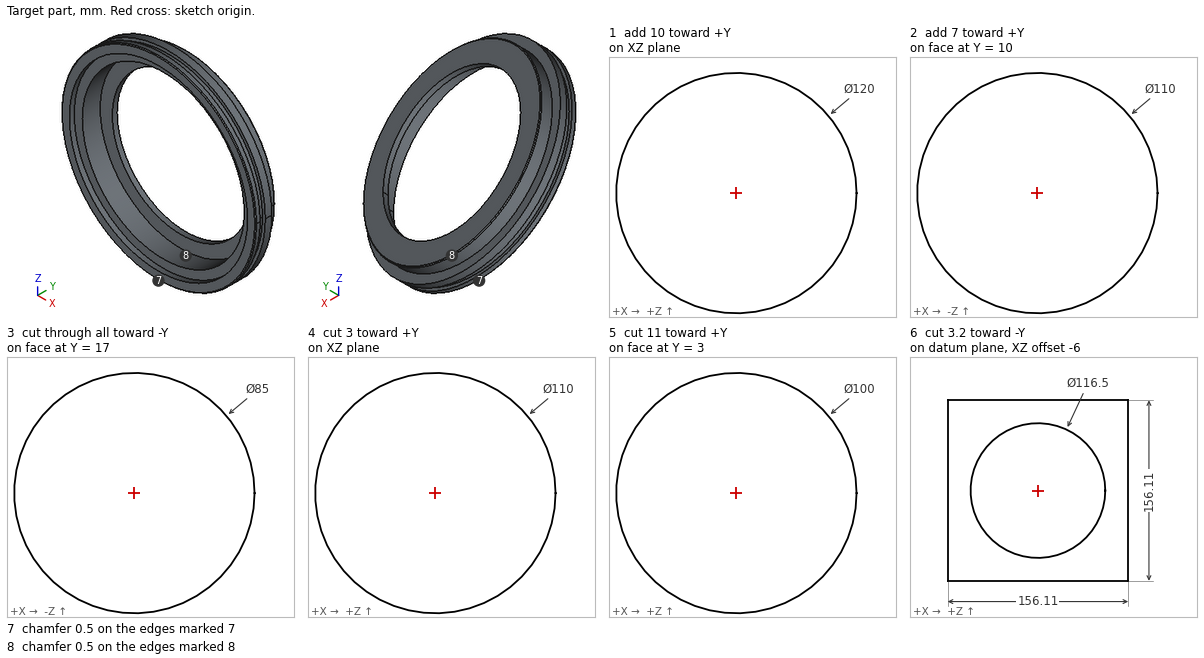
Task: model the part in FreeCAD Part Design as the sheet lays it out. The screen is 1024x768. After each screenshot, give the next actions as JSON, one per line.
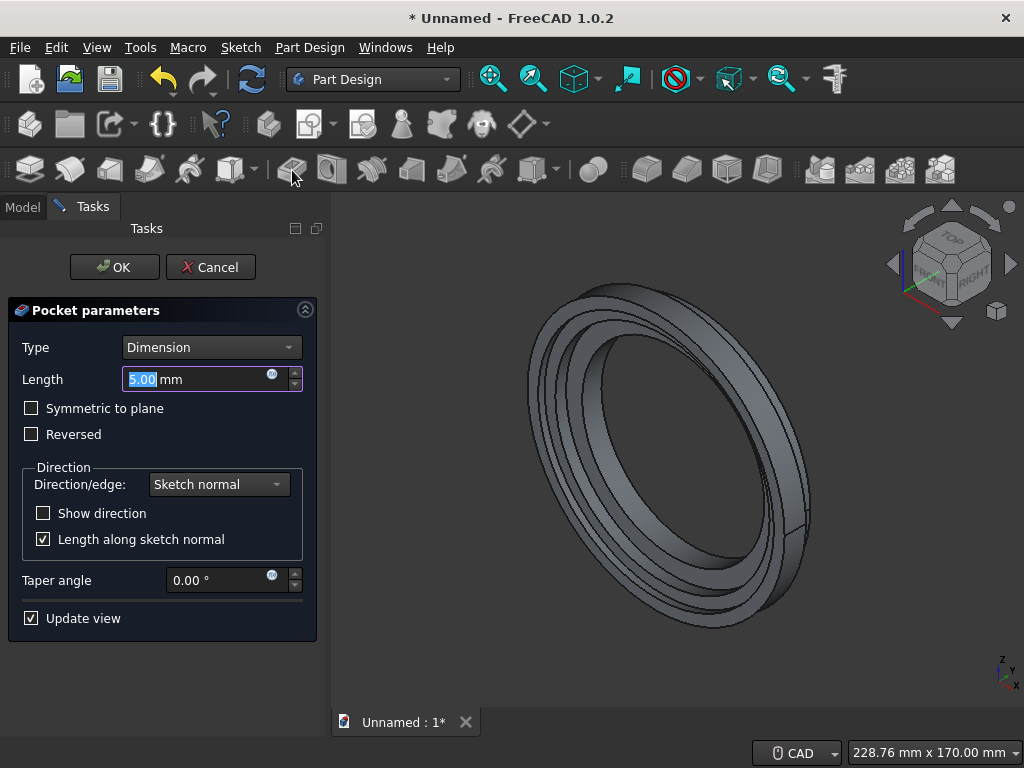
{"action": "type", "text": "11"}
{"action": "key", "text": "Tab"}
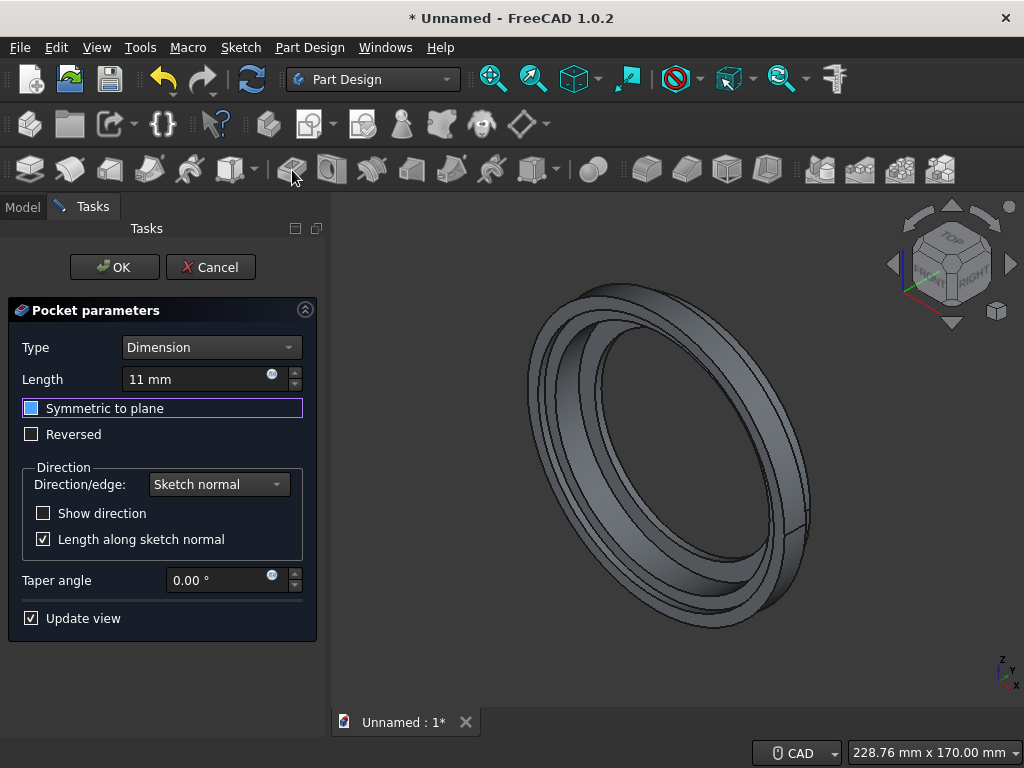
{"action": "left_click", "coordinate": [115, 267]}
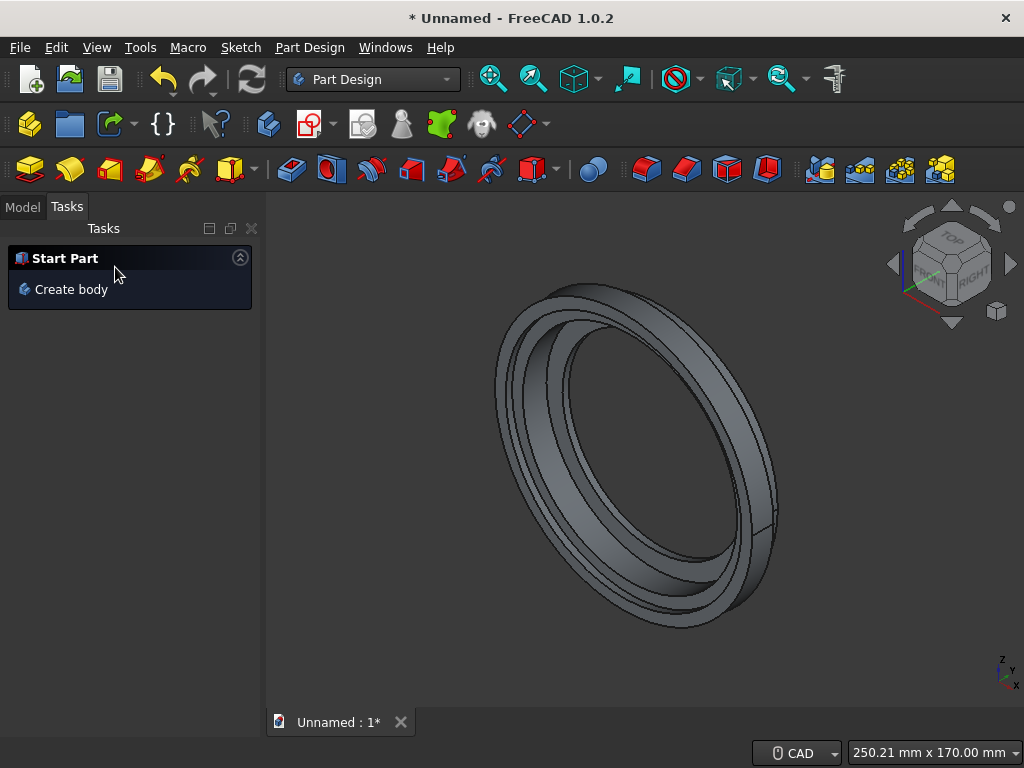
{"action": "left_click", "coordinate": [23, 206]}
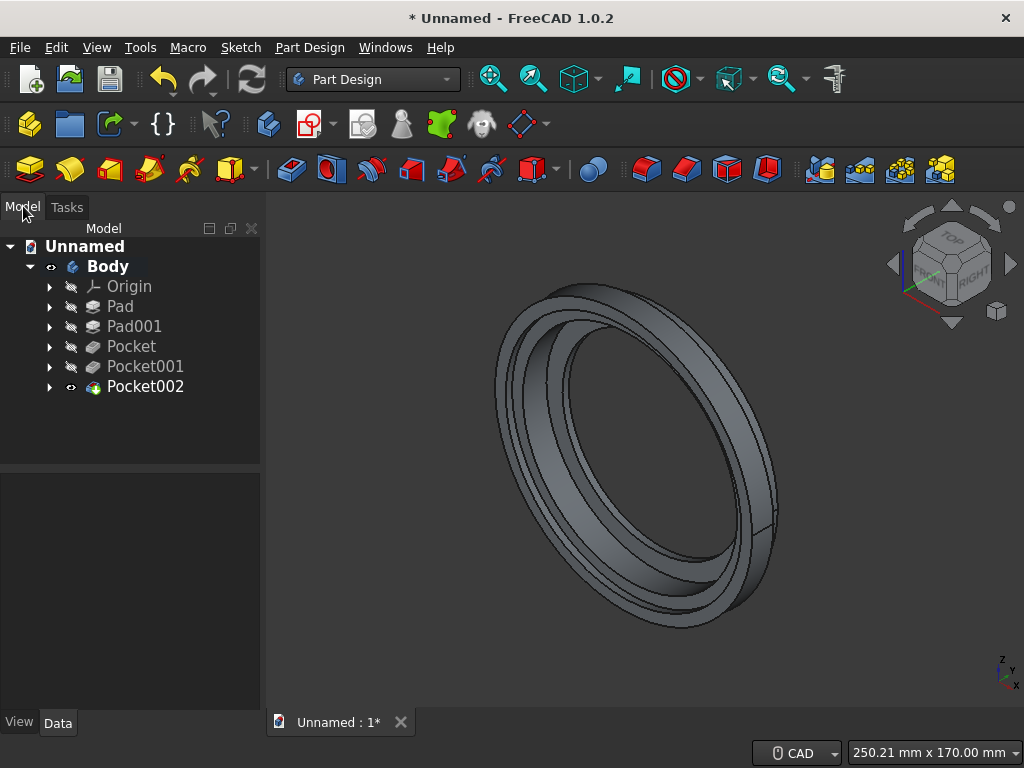
{"action": "left_click", "coordinate": [50, 287]}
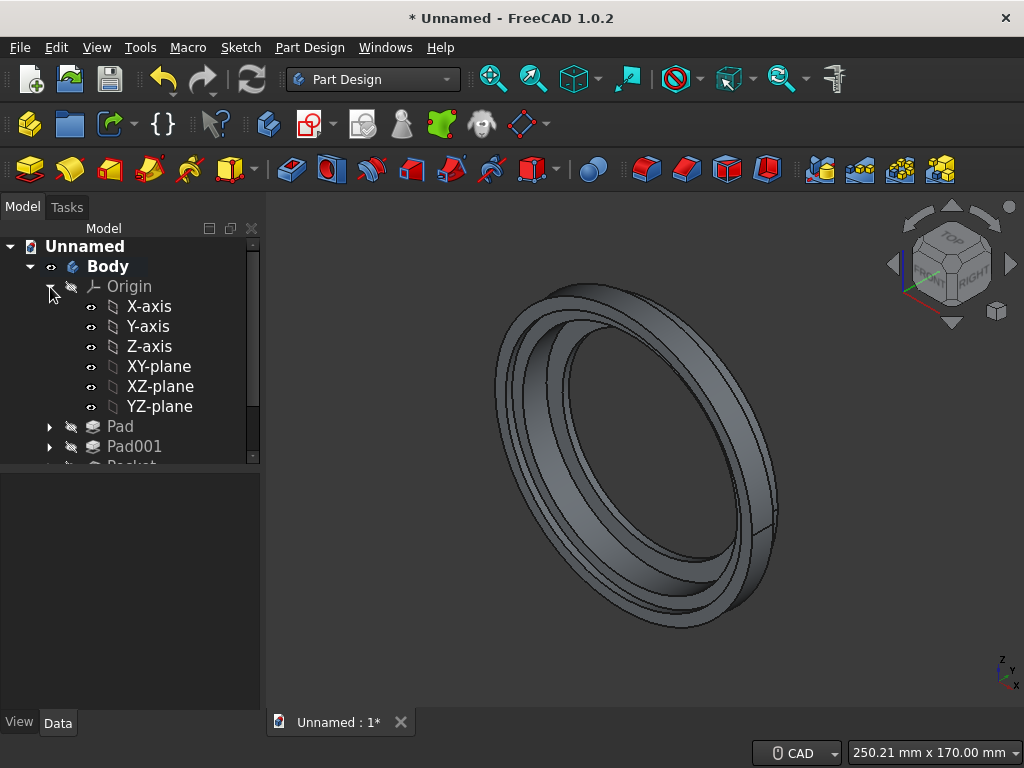
{"action": "left_click", "coordinate": [136, 387]}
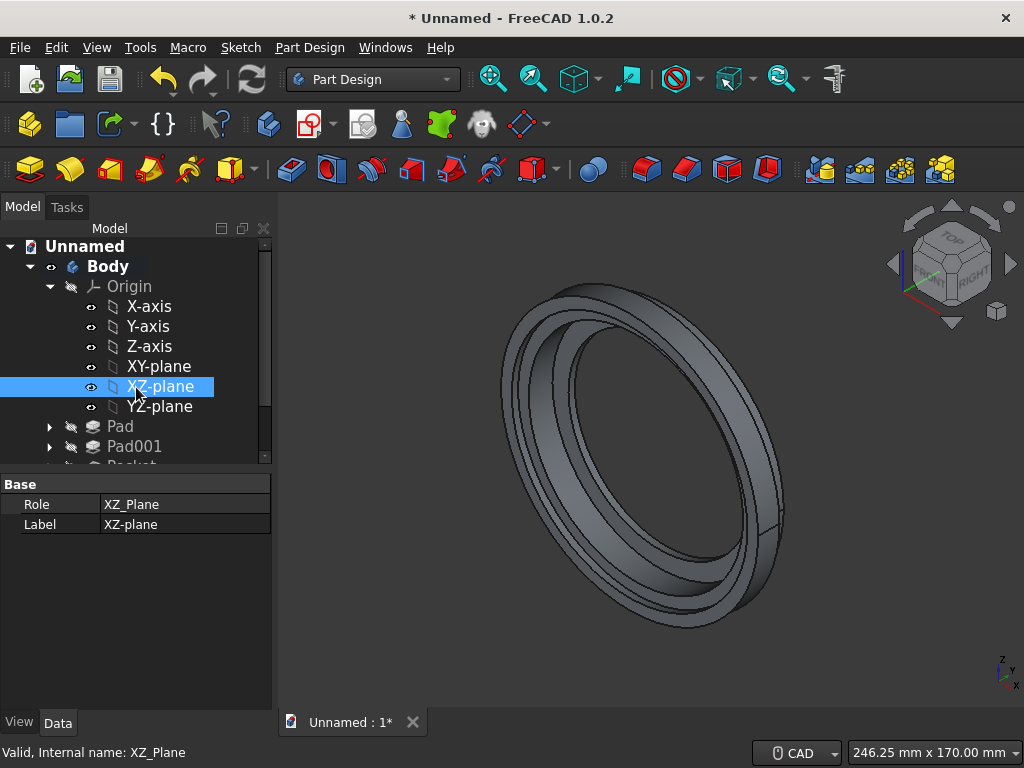
{"action": "left_click", "coordinate": [522, 124]}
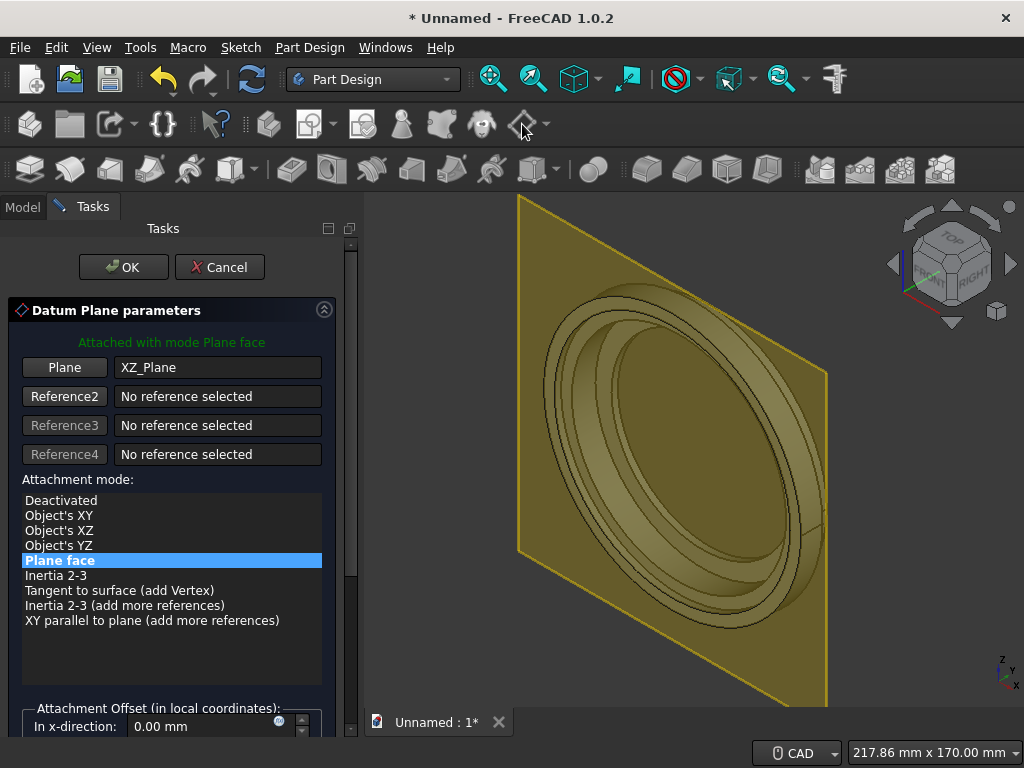
{"action": "scroll", "coordinate": [351, 487], "scroll_direction": "down", "scroll_amount": 3}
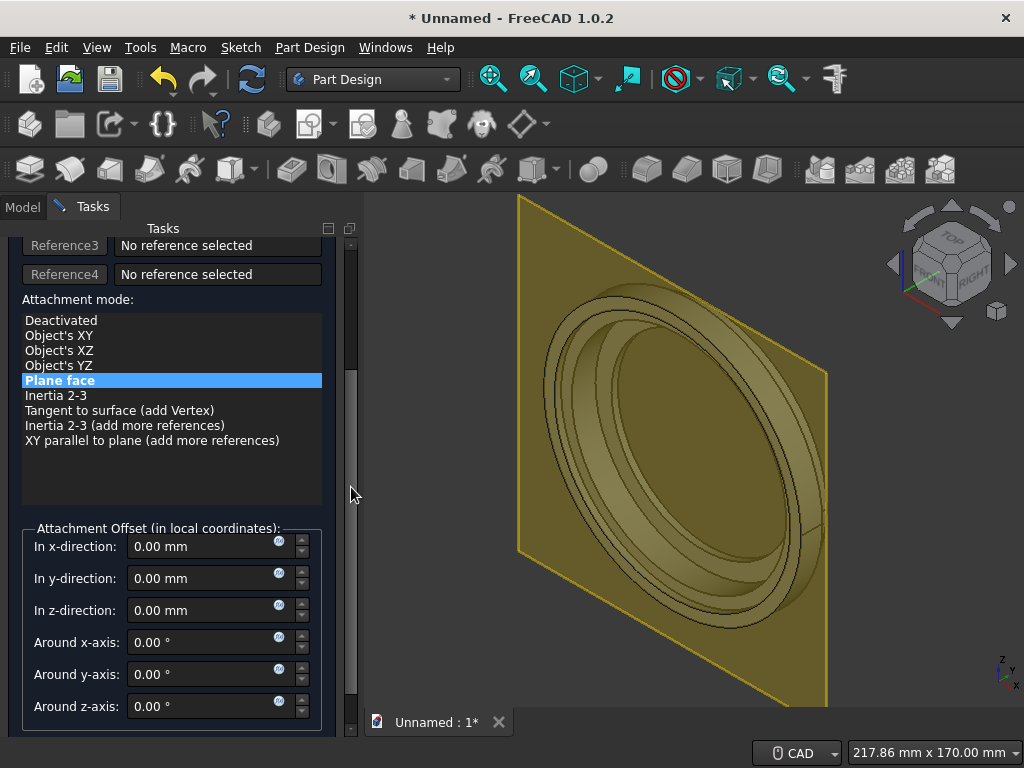
{"action": "triple_click", "coordinate": [210, 610]}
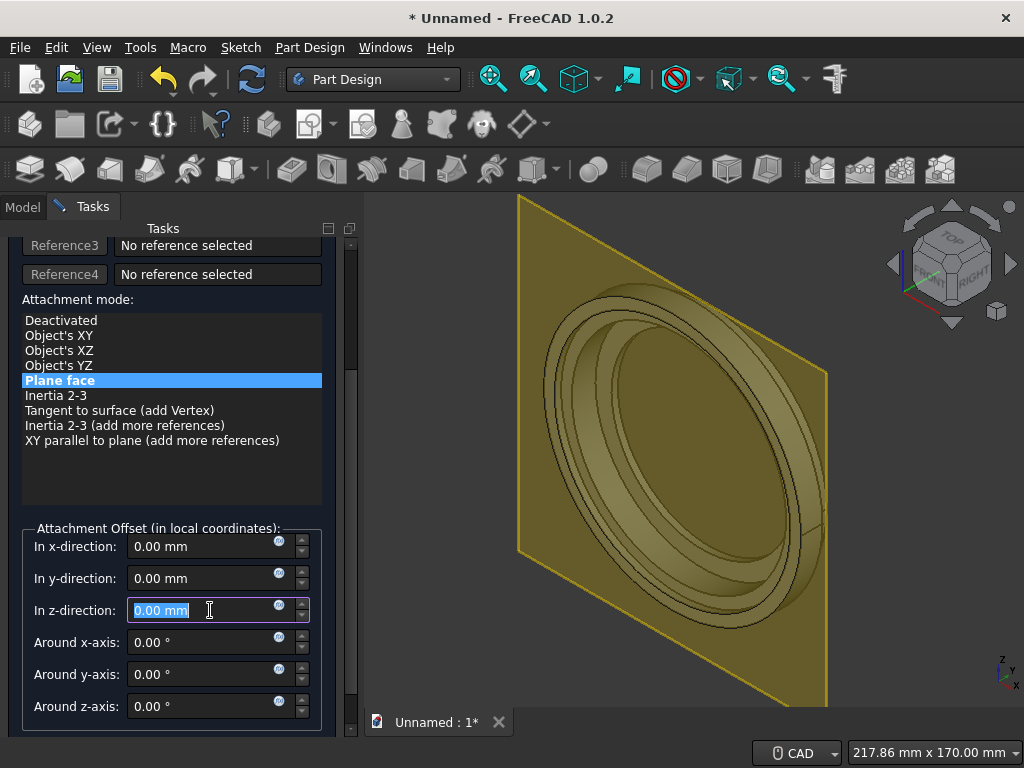
{"action": "type", "text": "-6"}
{"action": "key", "text": "Tab"}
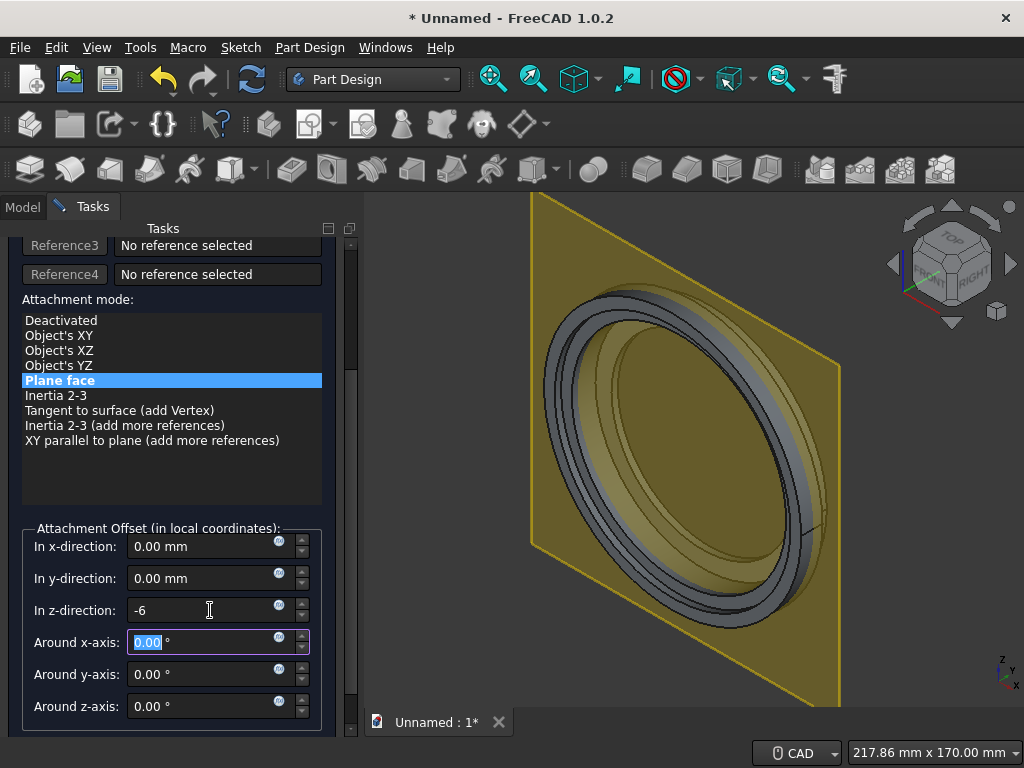
{"action": "scroll", "coordinate": [351, 487], "scroll_direction": "up", "scroll_amount": 4}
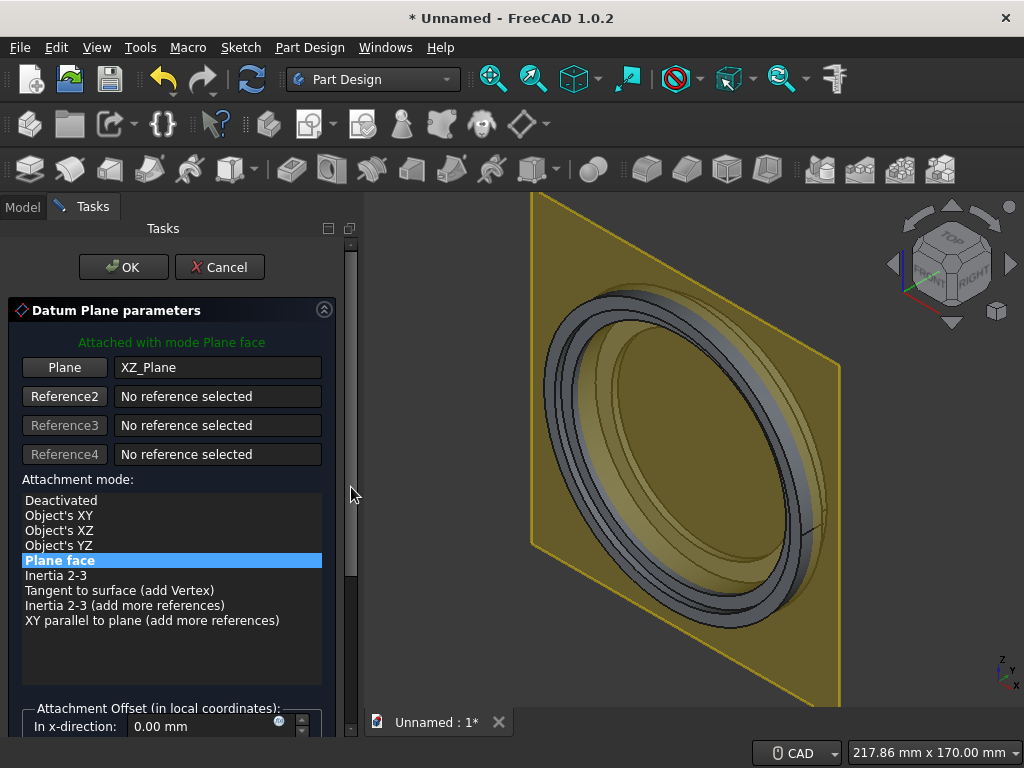
{"action": "left_click", "coordinate": [124, 267]}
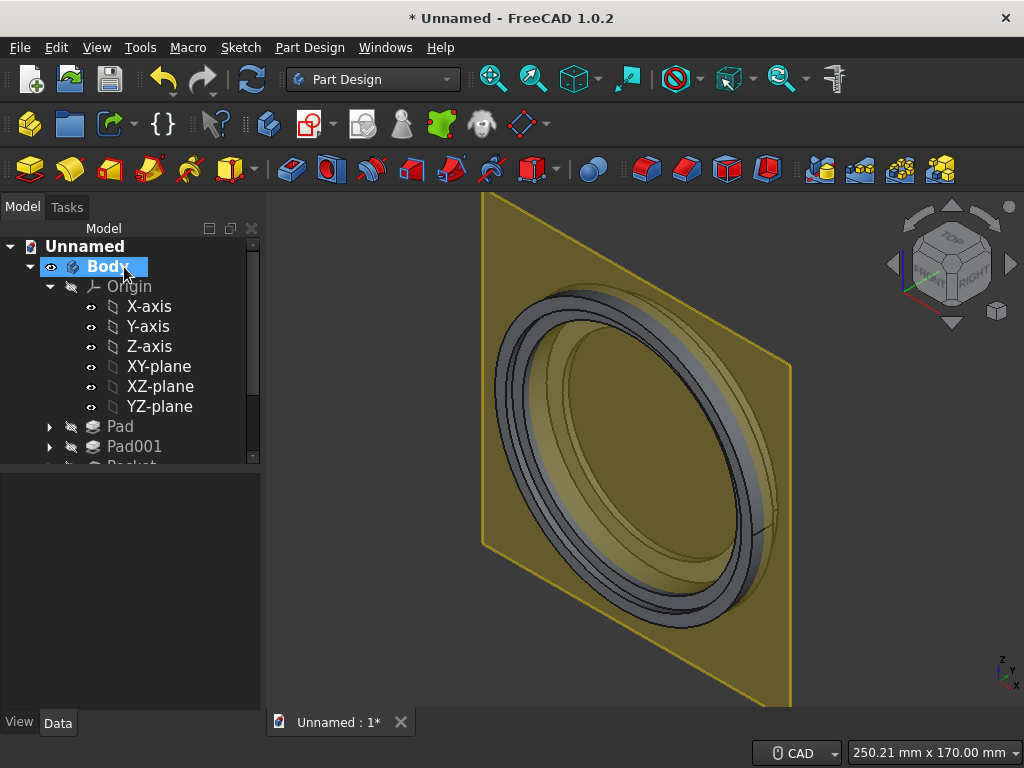
{"action": "scroll", "coordinate": [100, 342], "scroll_direction": "down", "scroll_amount": 3}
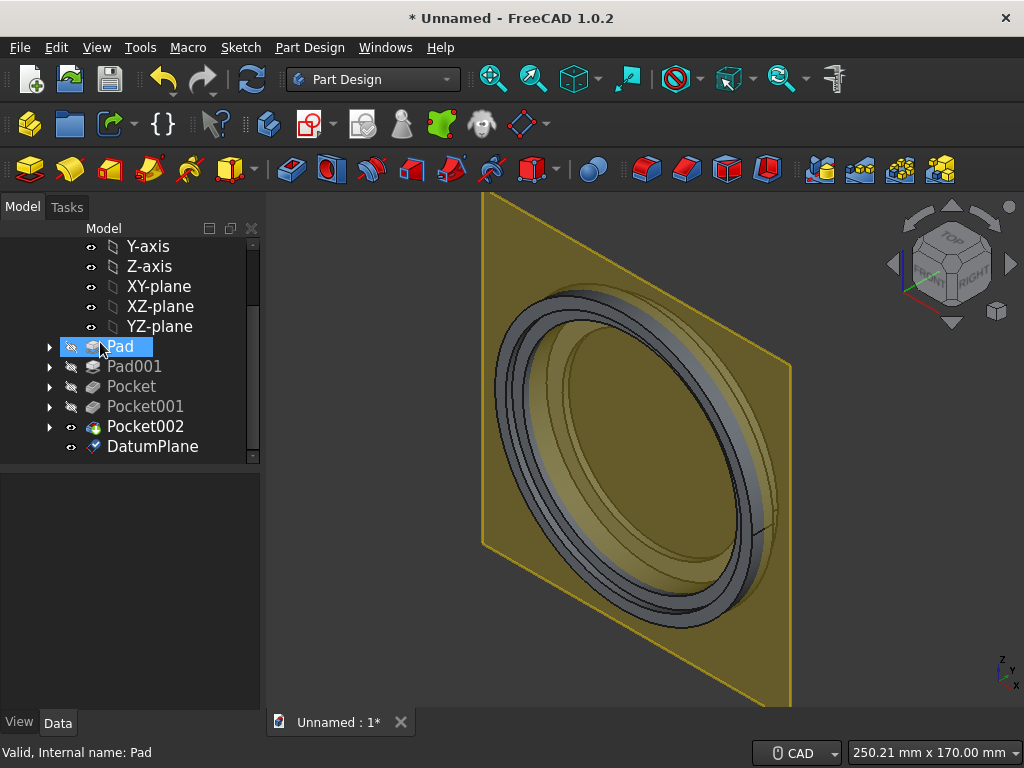
{"action": "left_click", "coordinate": [116, 447]}